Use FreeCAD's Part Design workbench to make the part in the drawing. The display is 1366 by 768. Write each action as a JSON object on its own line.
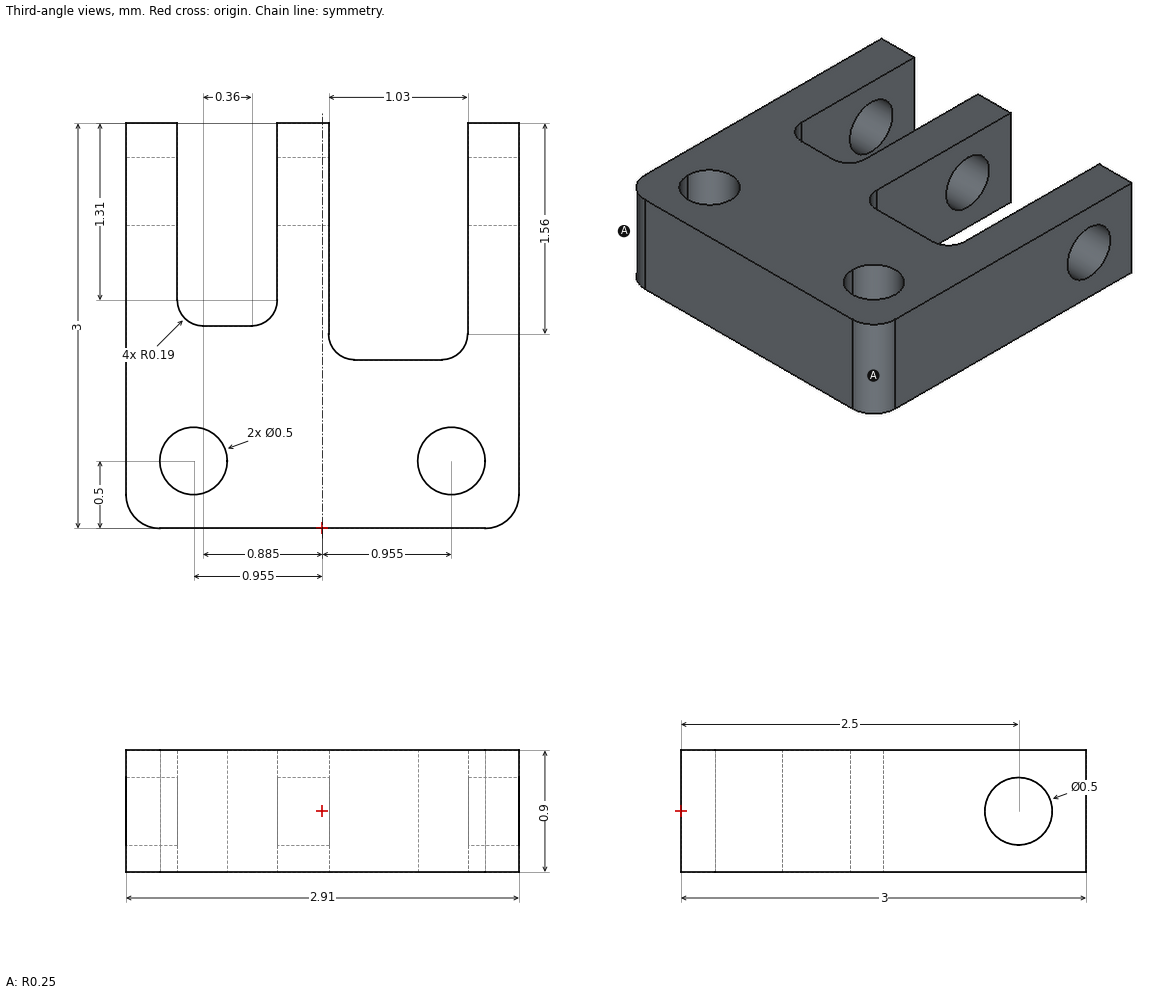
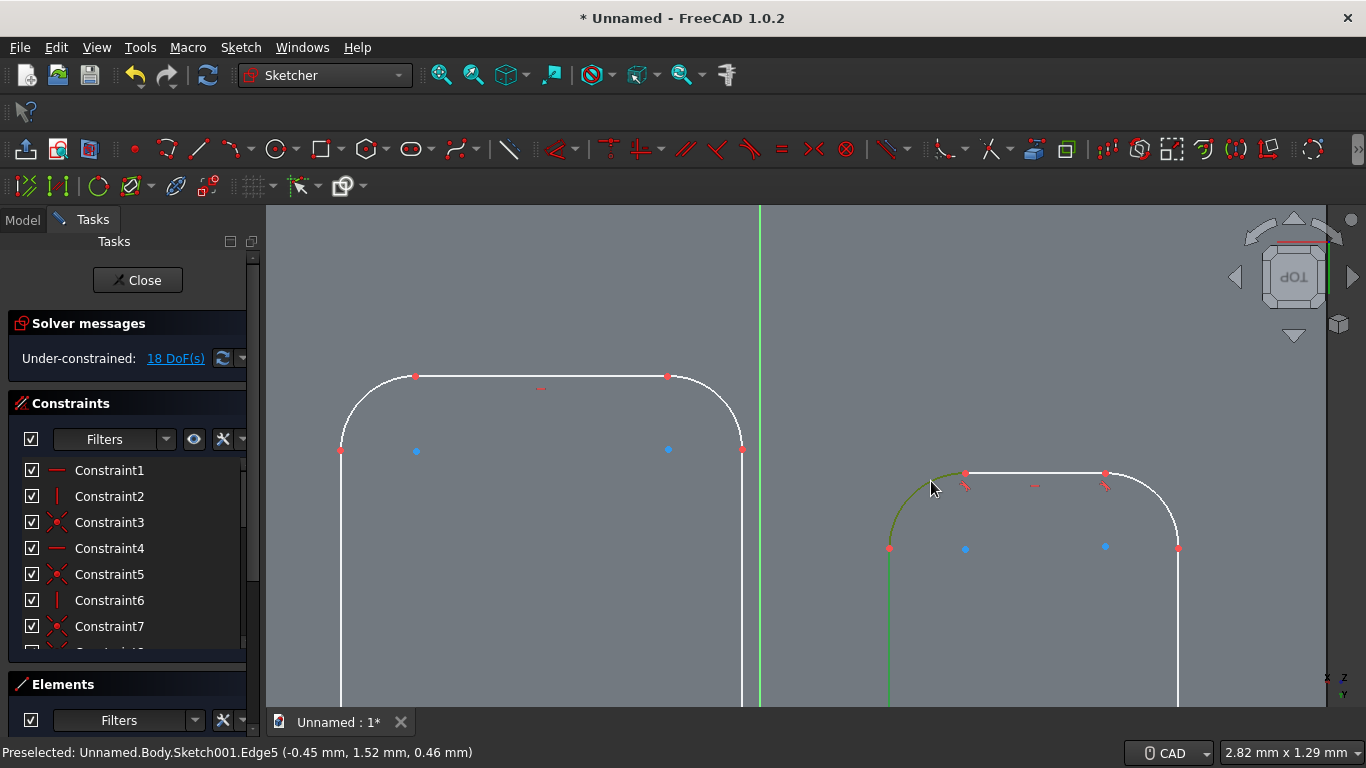
{"action": "key", "text": "t"}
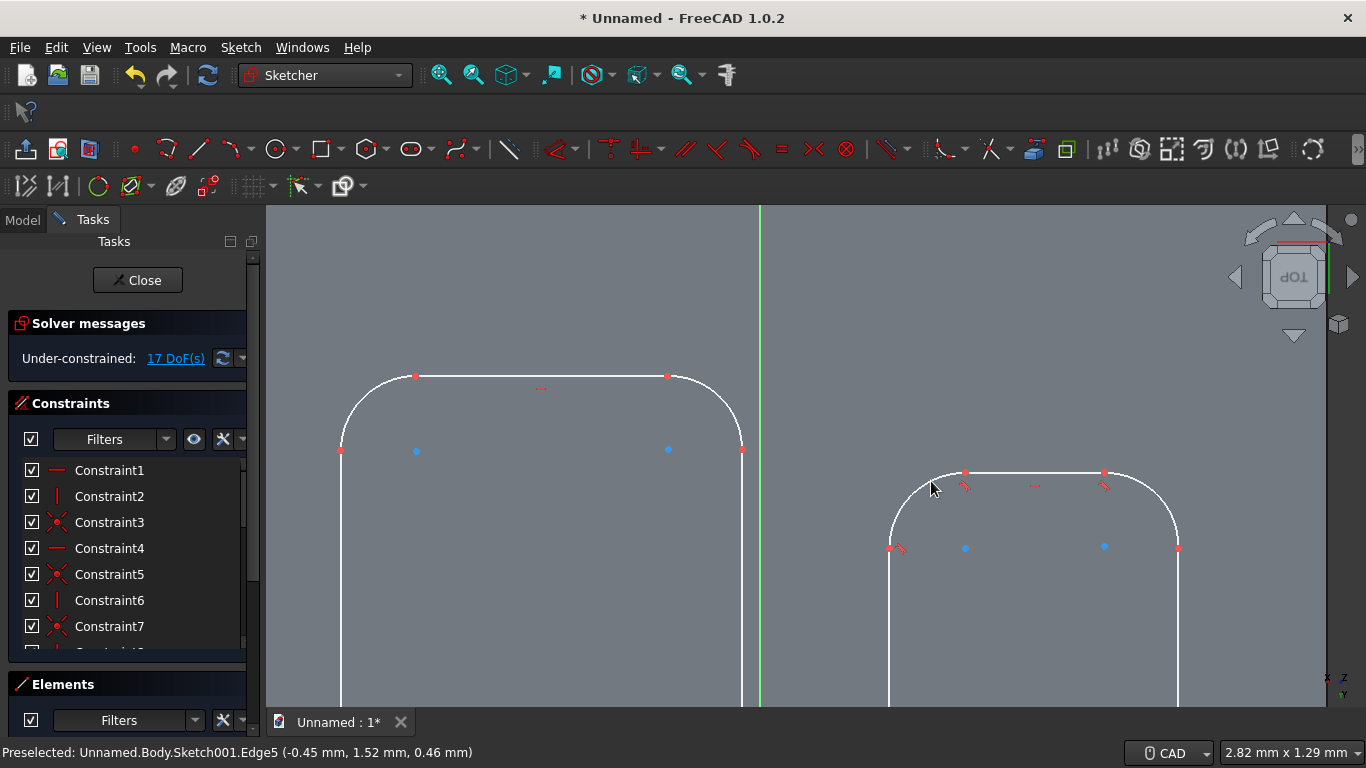
{"action": "left_click", "coordinate": [1178, 651]}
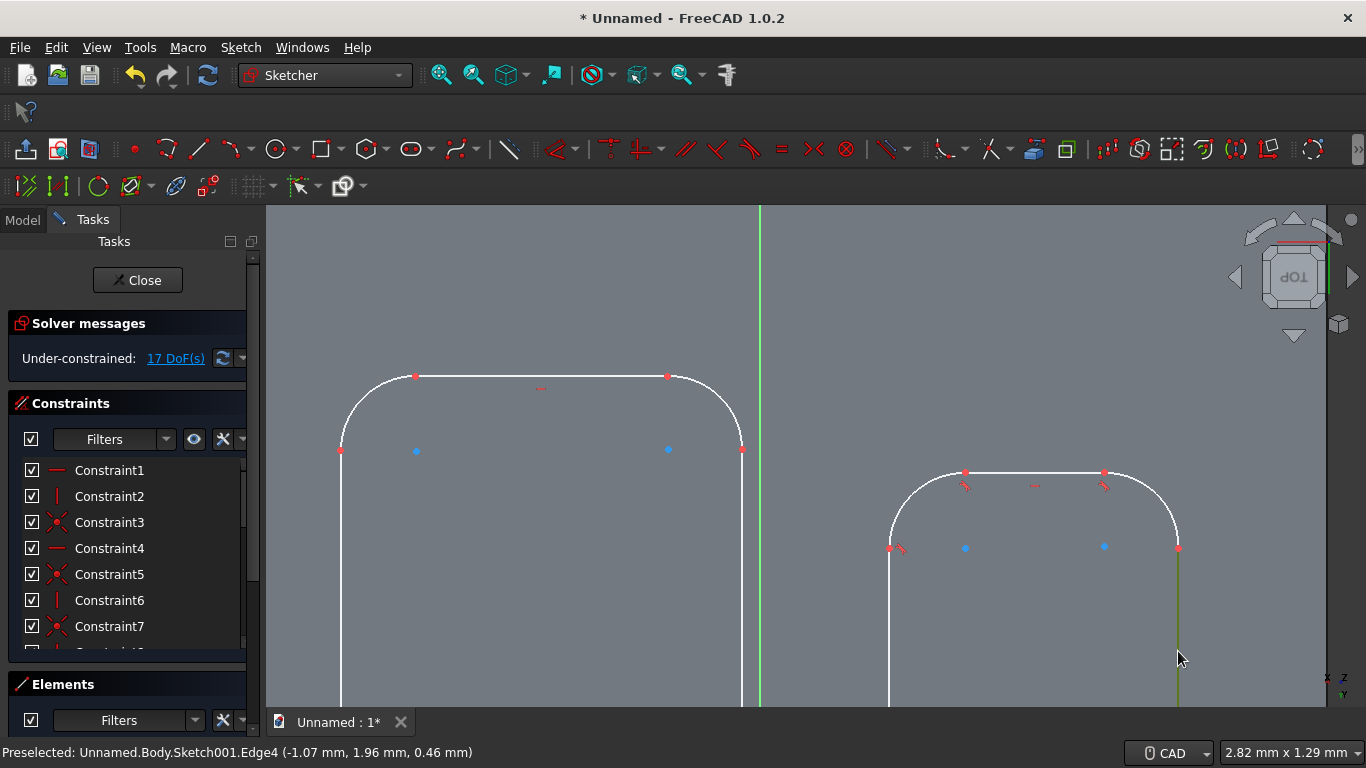
{"action": "left_click", "coordinate": [1171, 515]}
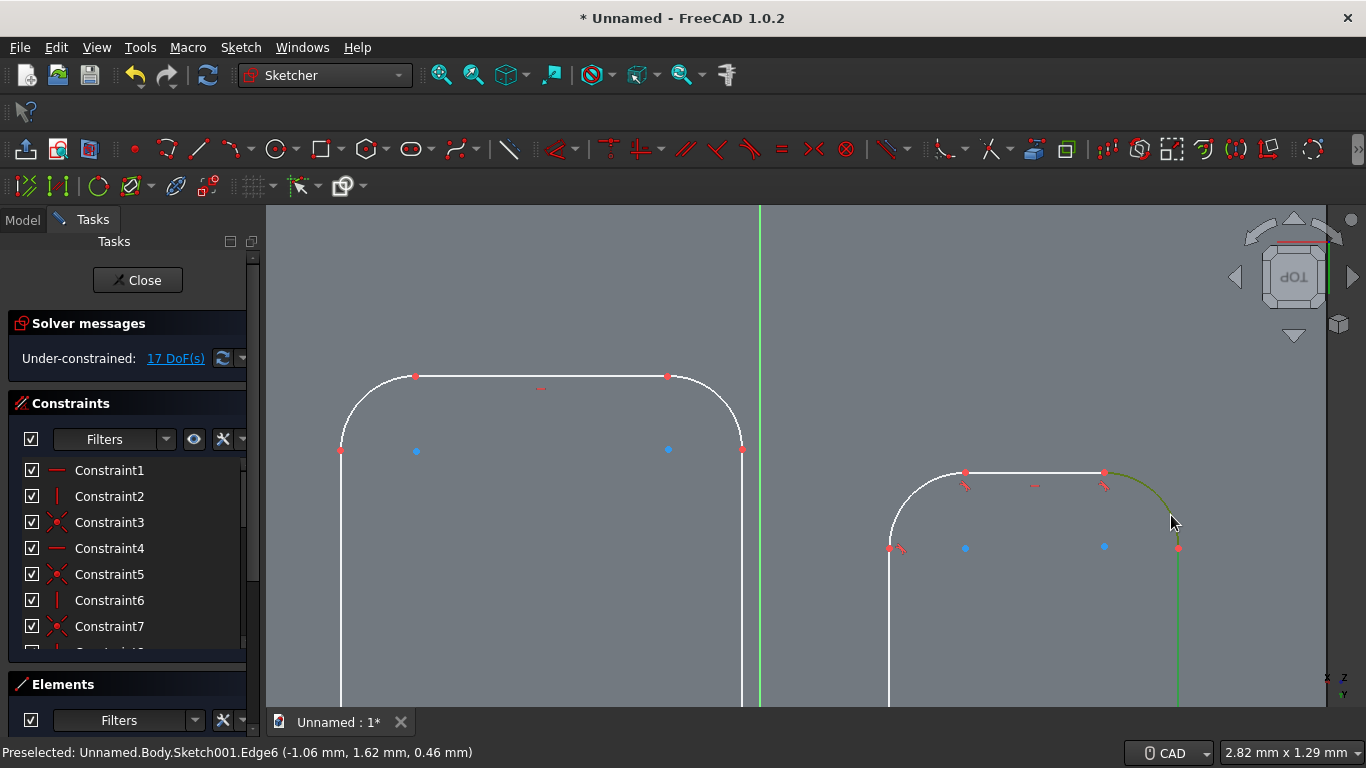
{"action": "key", "text": "t"}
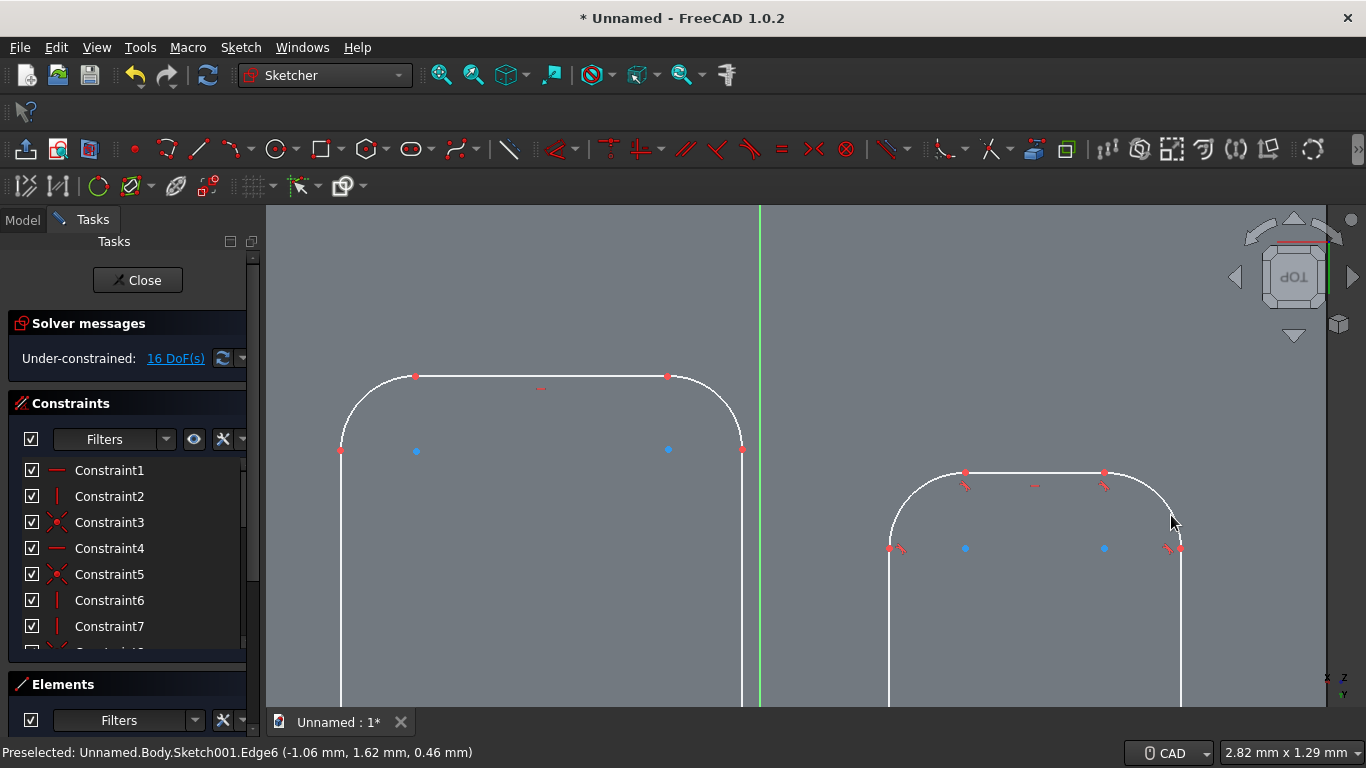
{"action": "left_click", "coordinate": [341, 634]}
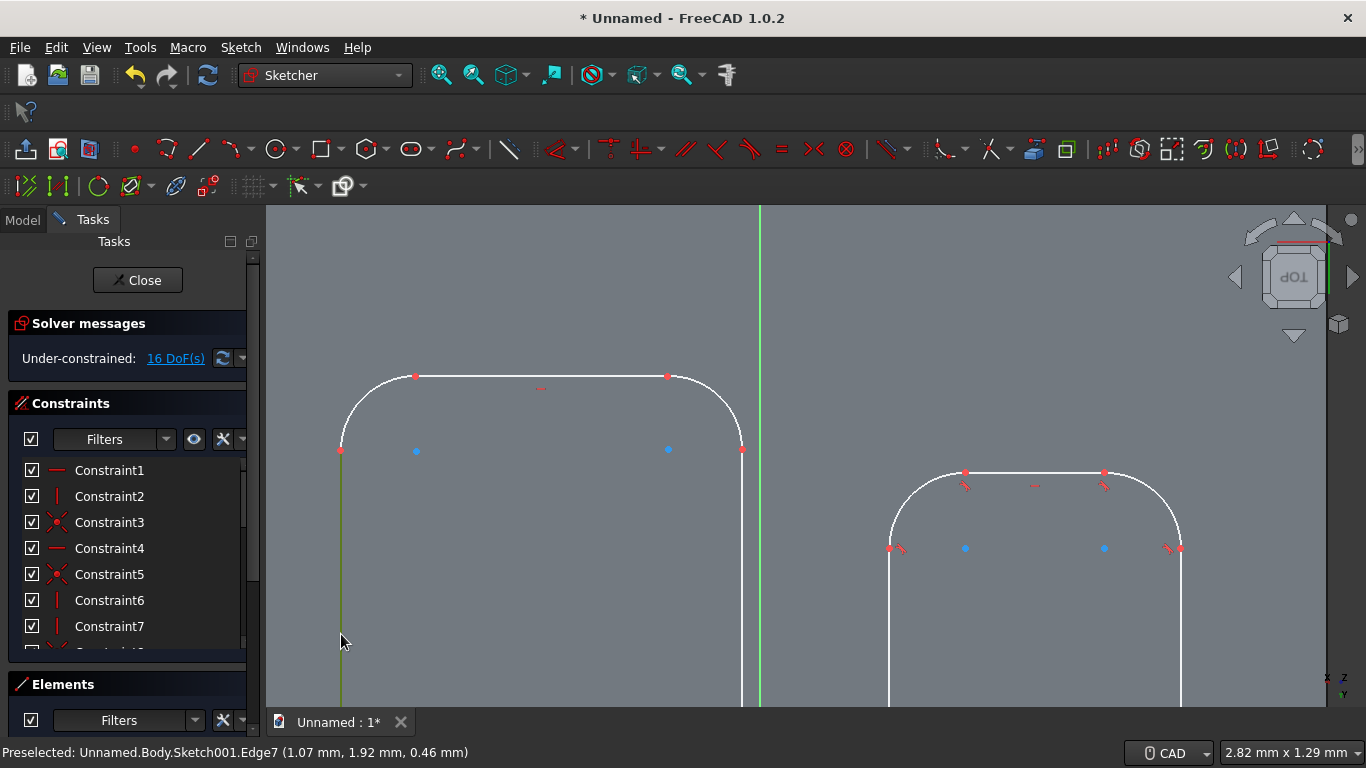
{"action": "left_click", "coordinate": [382, 384]}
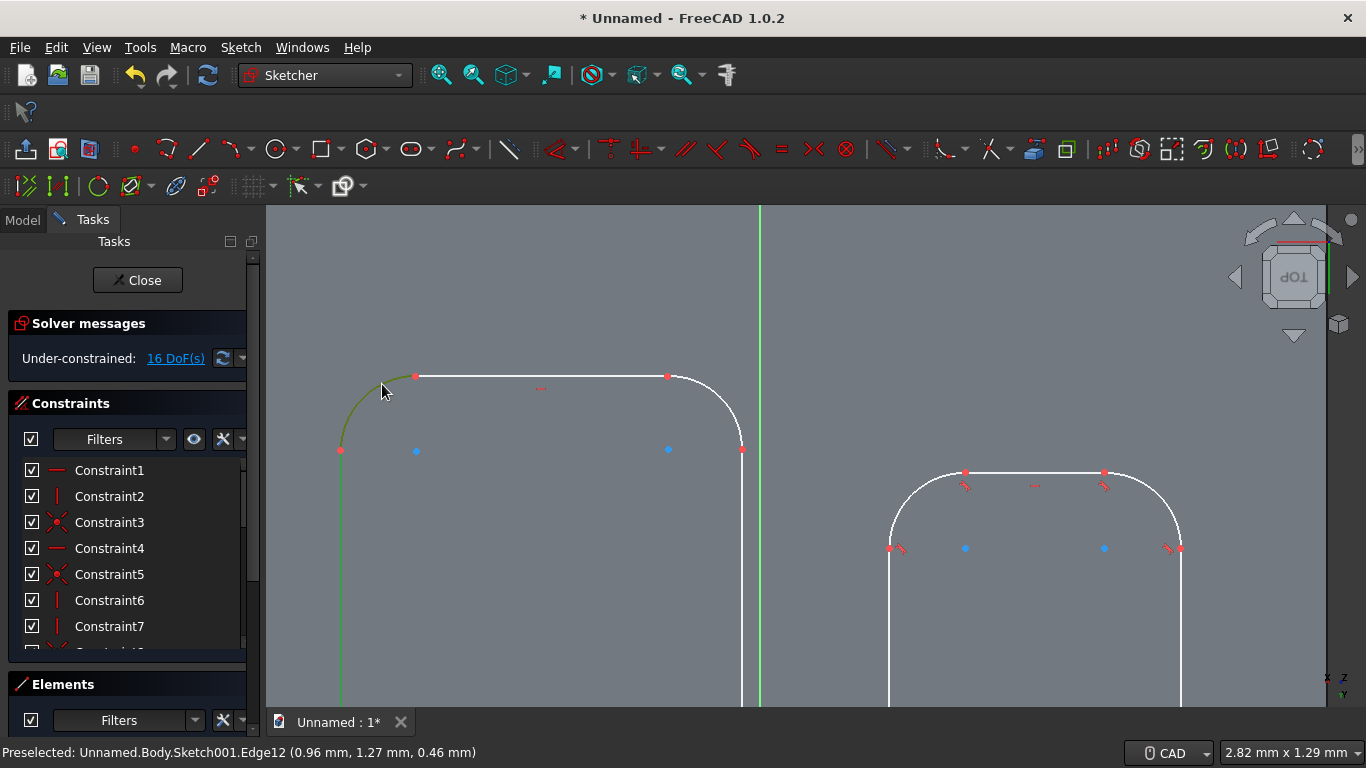
{"action": "key", "text": "t"}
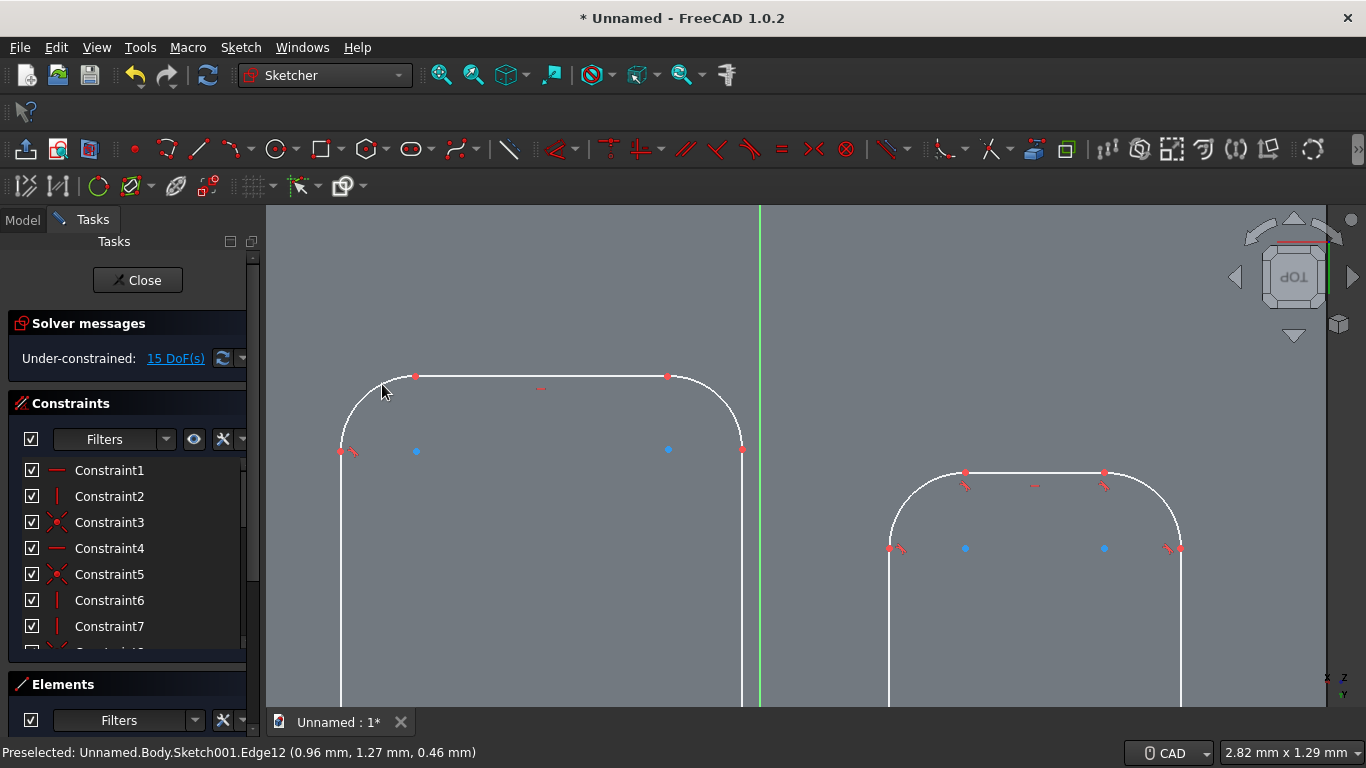
{"action": "left_click", "coordinate": [742, 634]}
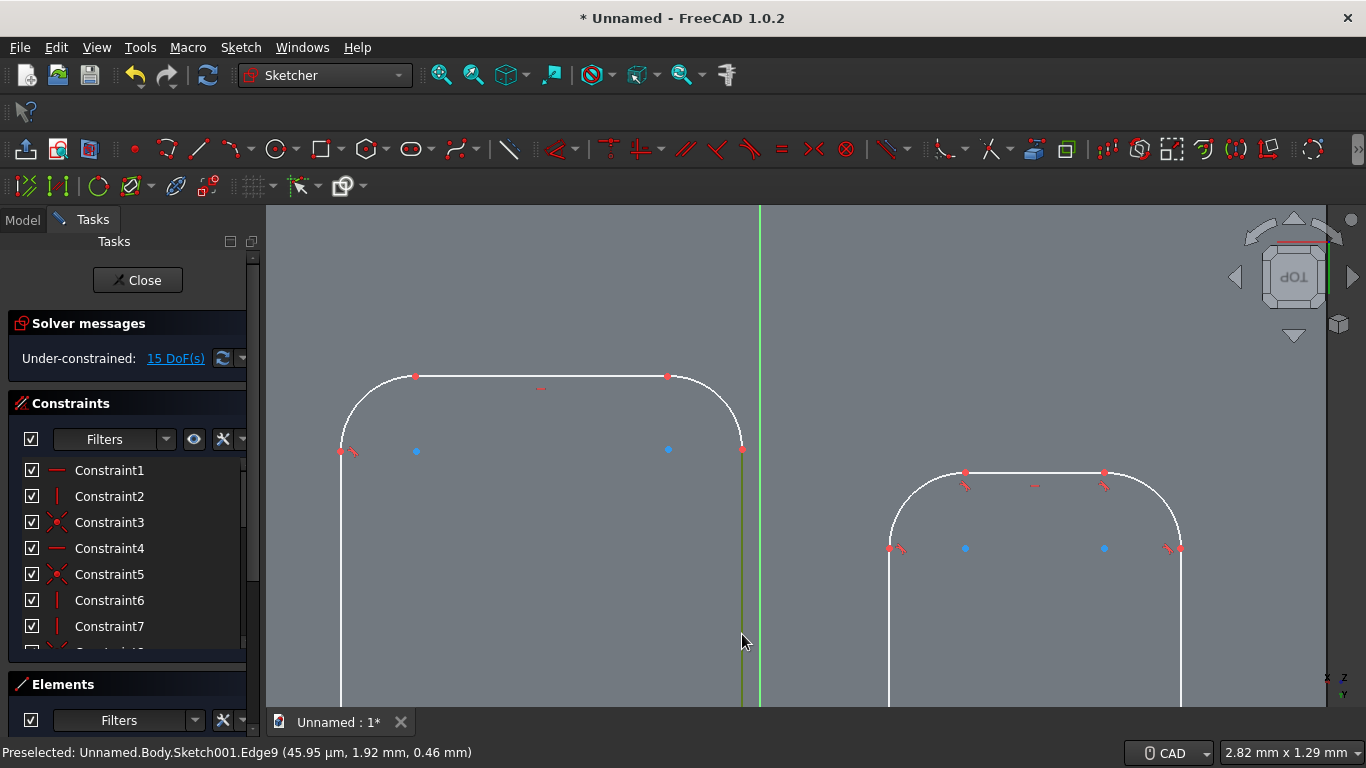
{"action": "left_click", "coordinate": [734, 416]}